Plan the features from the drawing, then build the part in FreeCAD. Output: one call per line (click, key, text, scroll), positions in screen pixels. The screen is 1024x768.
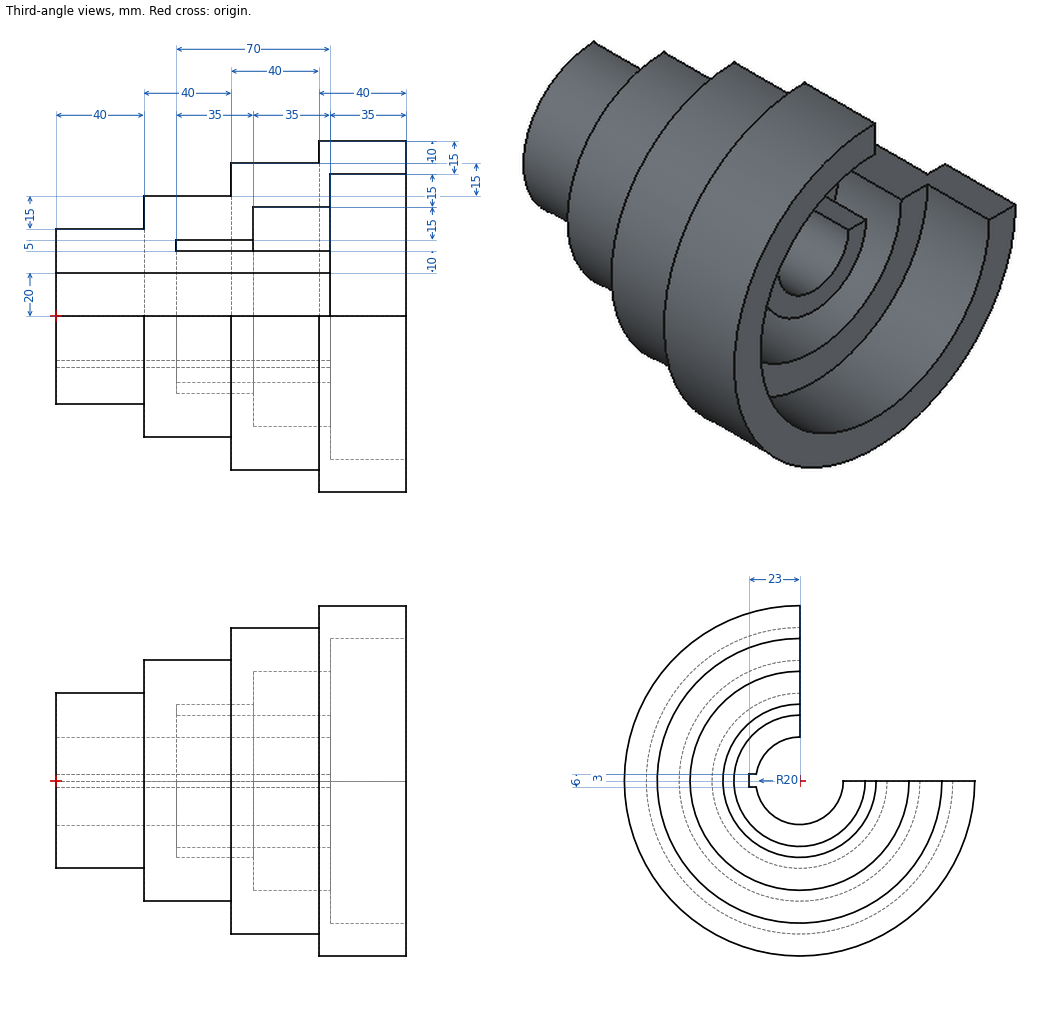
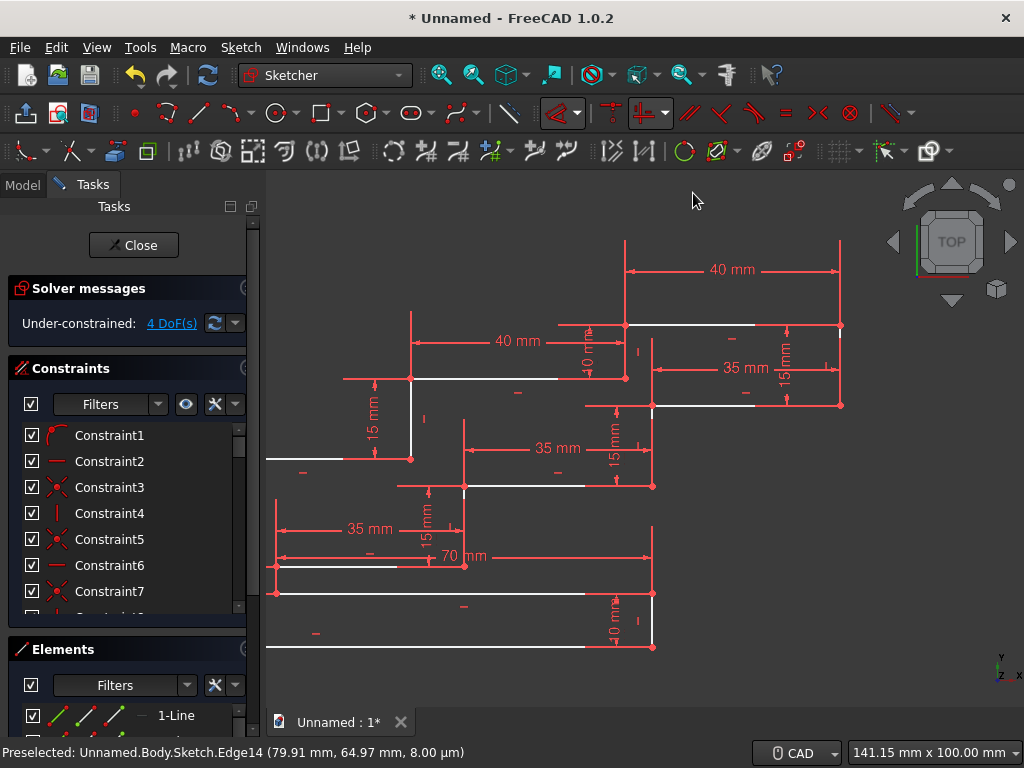
click(346, 459)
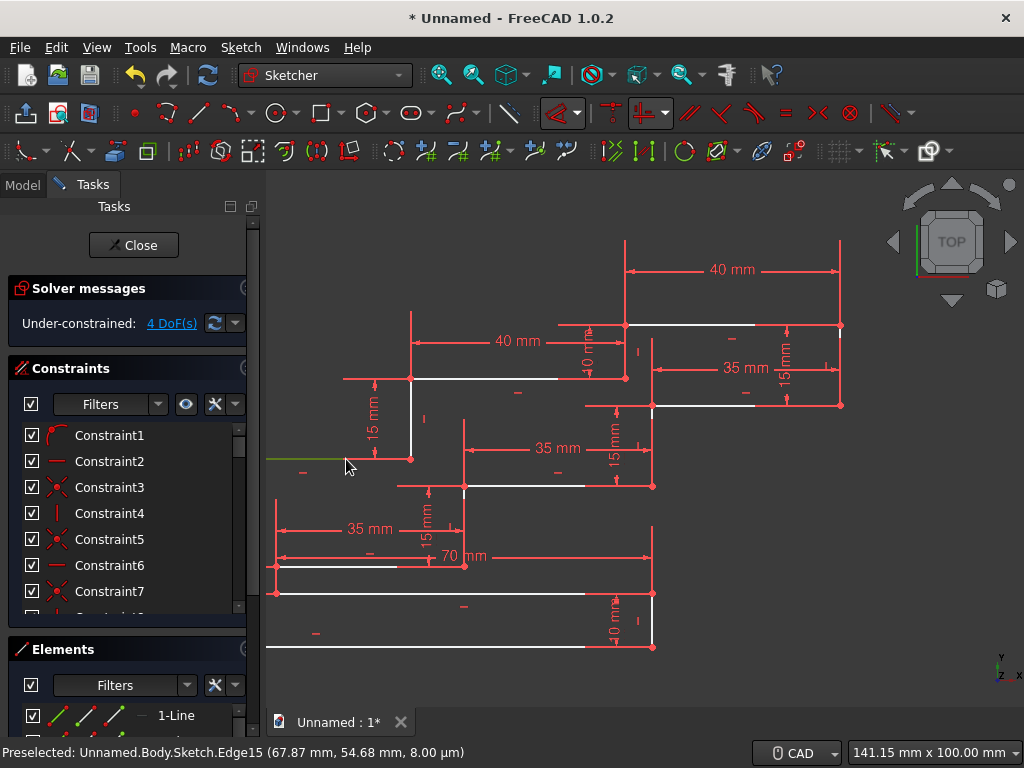
key(l)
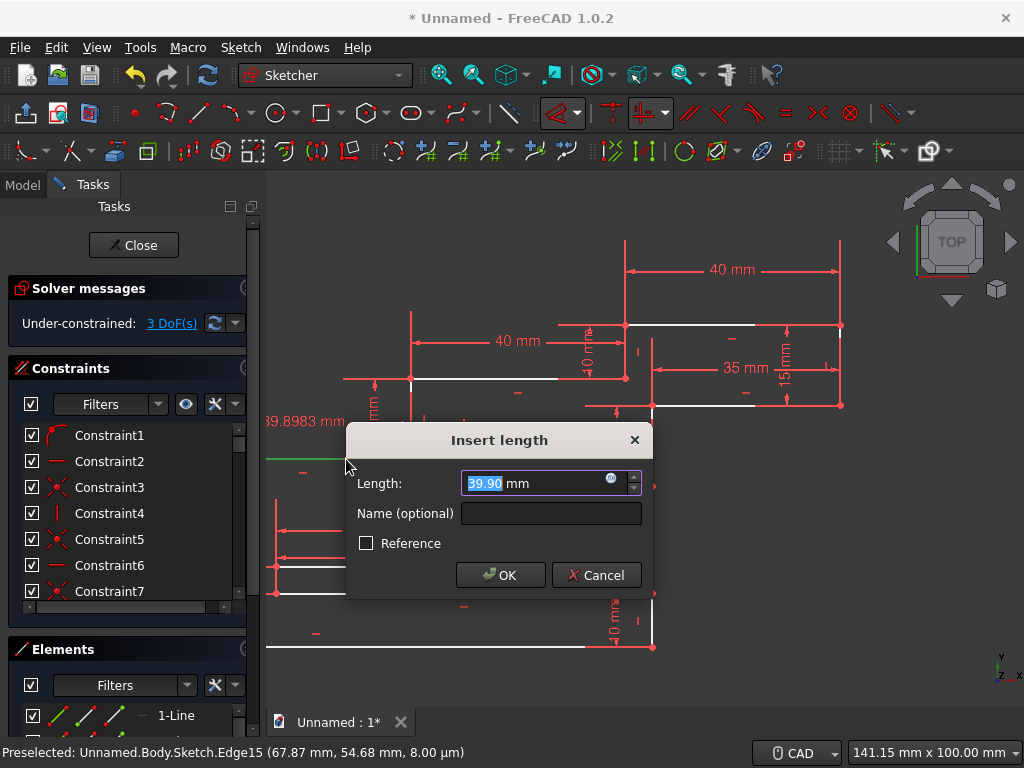
text(40)
key(Return)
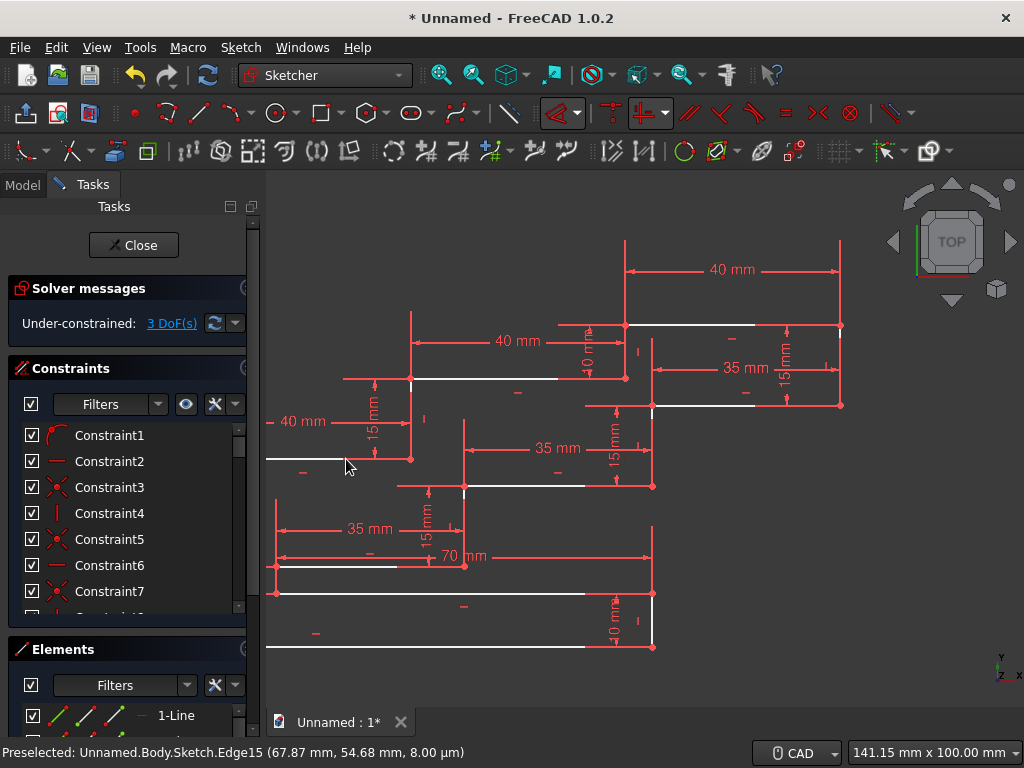
scroll(711, 357, down, 4)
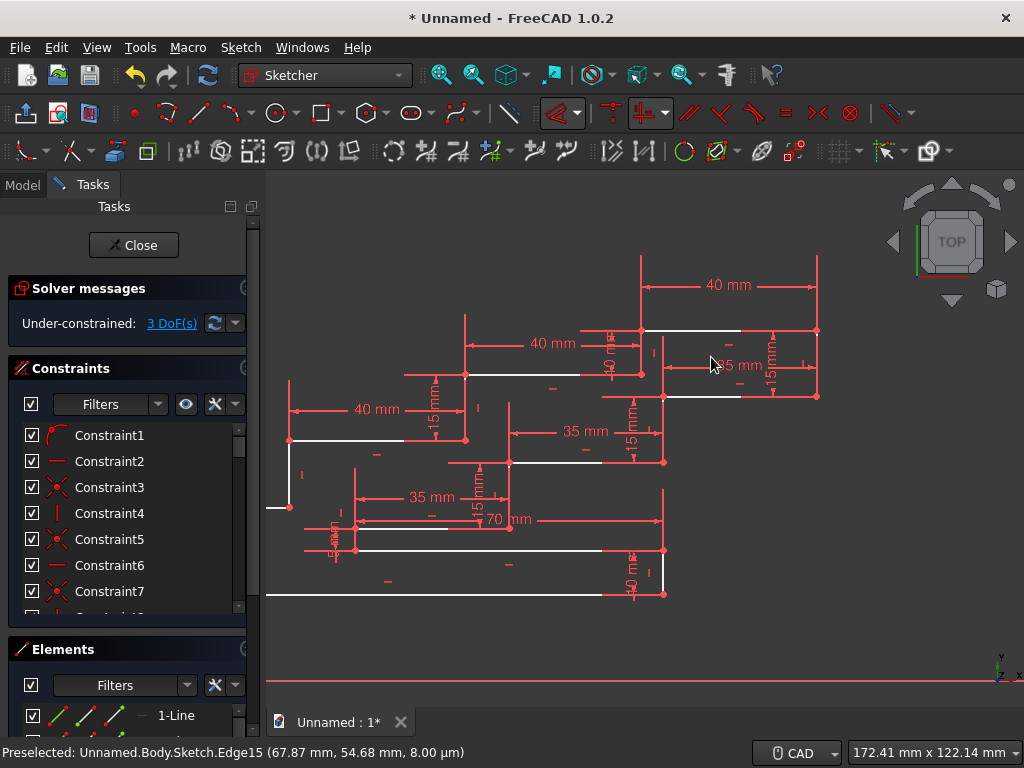
scroll(480, 414, up, 2)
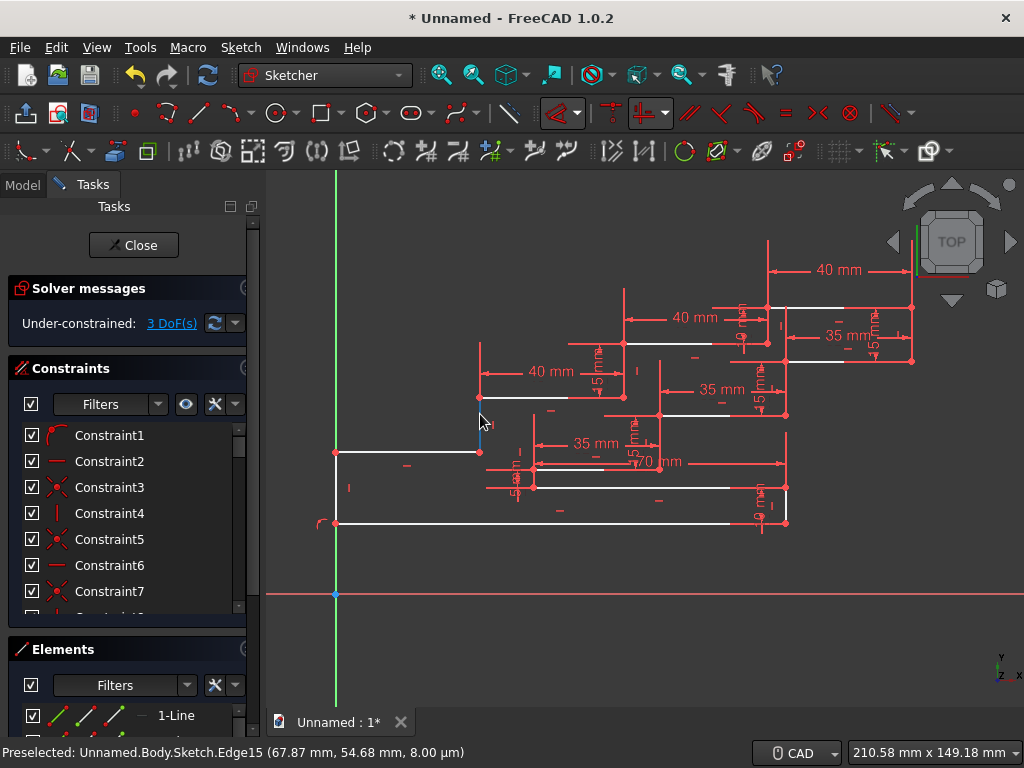
click(480, 414)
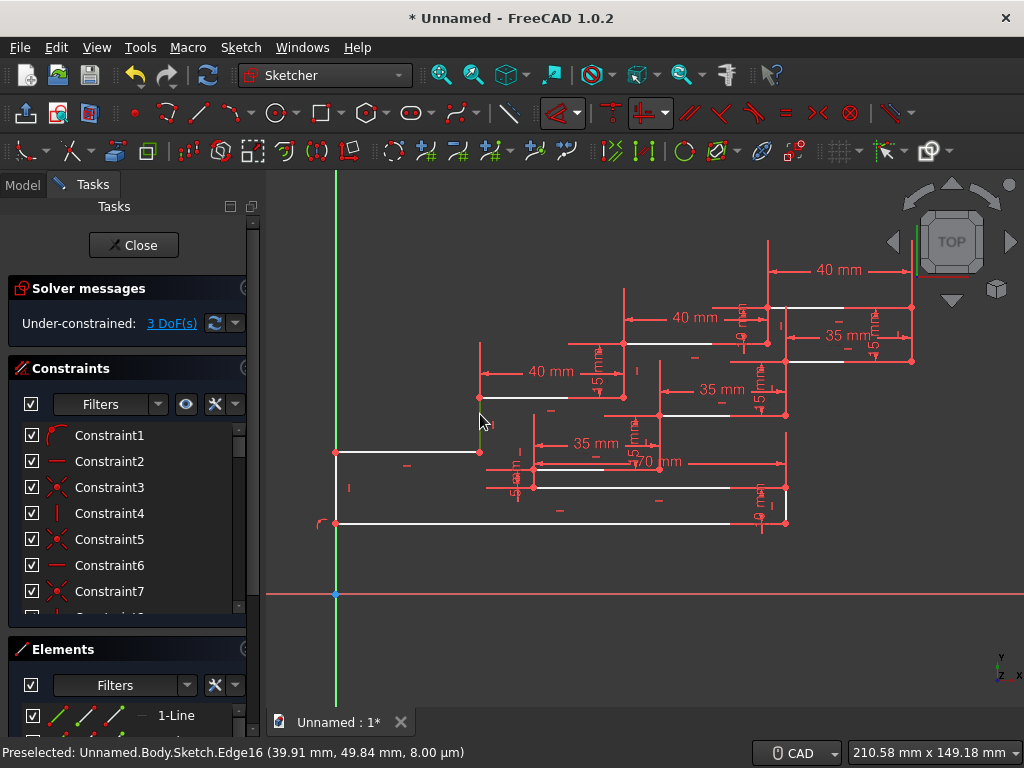
key(i)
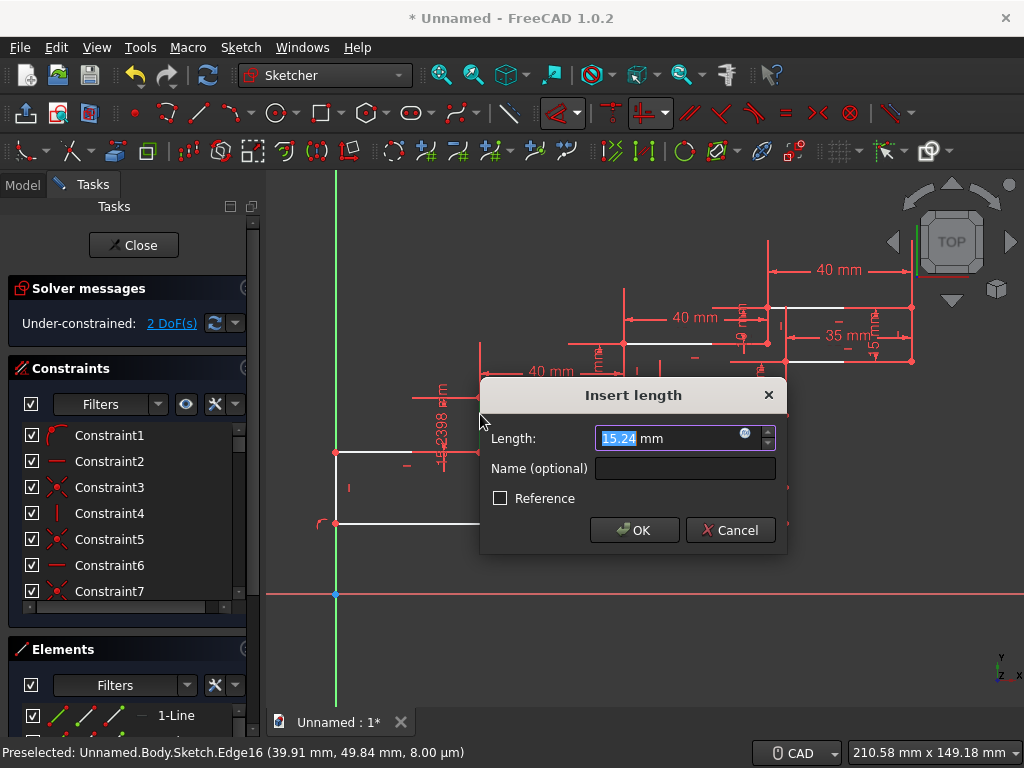
text(15)
key(Return)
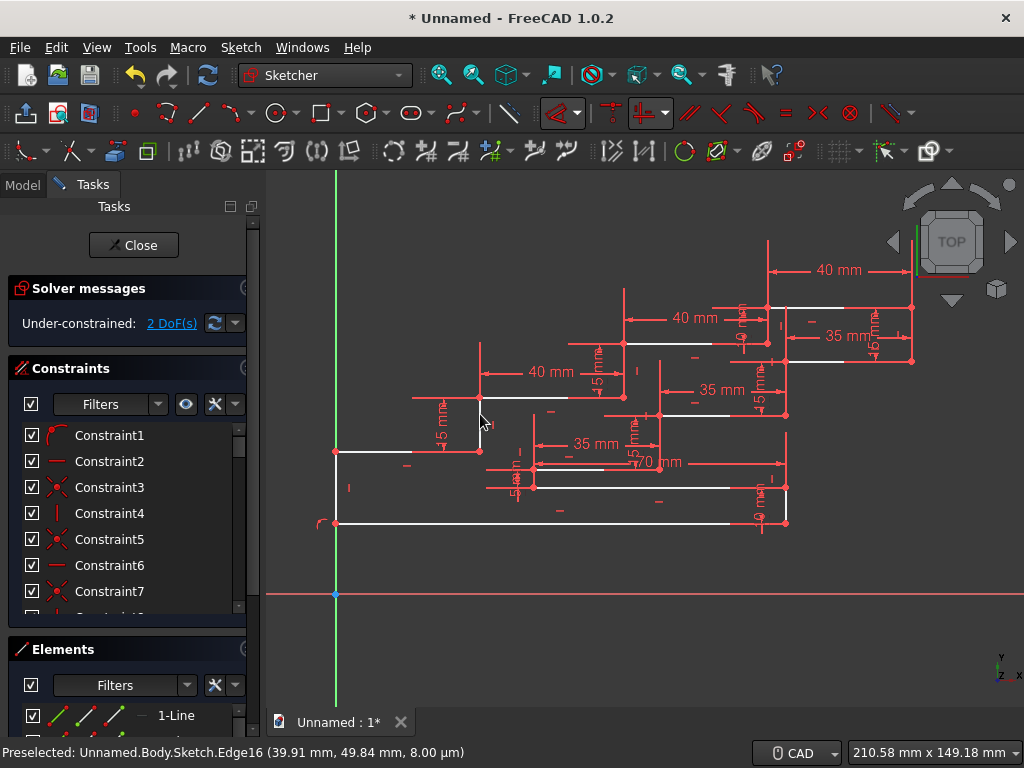
click(437, 452)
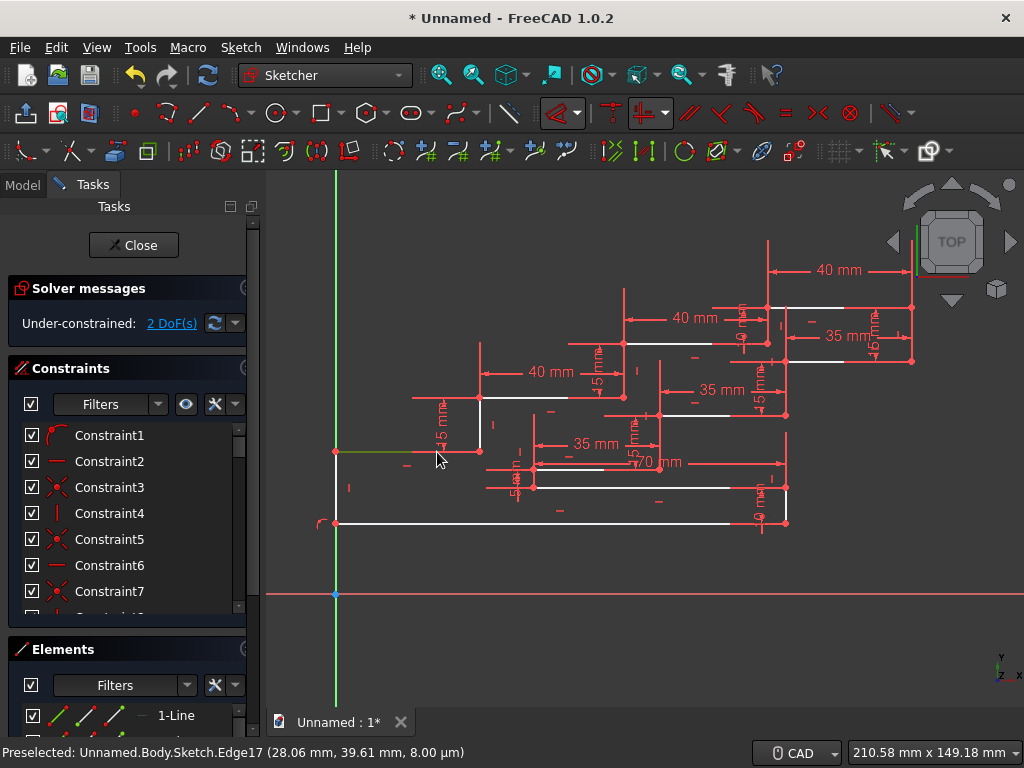
click(580, 114)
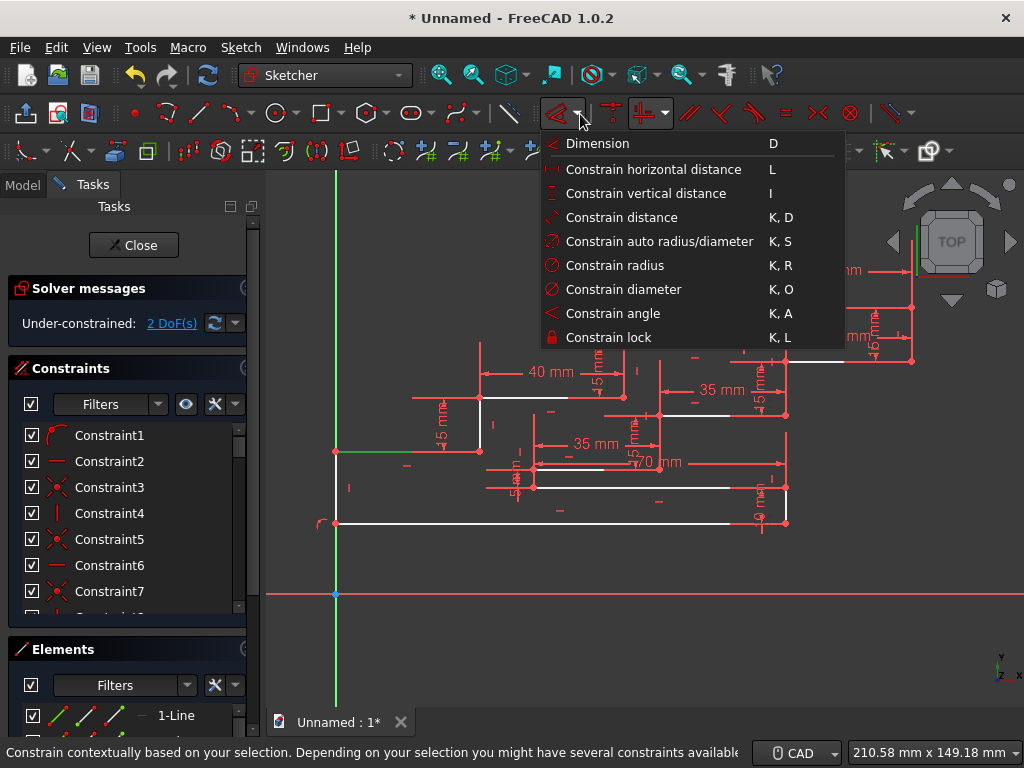
click(693, 169)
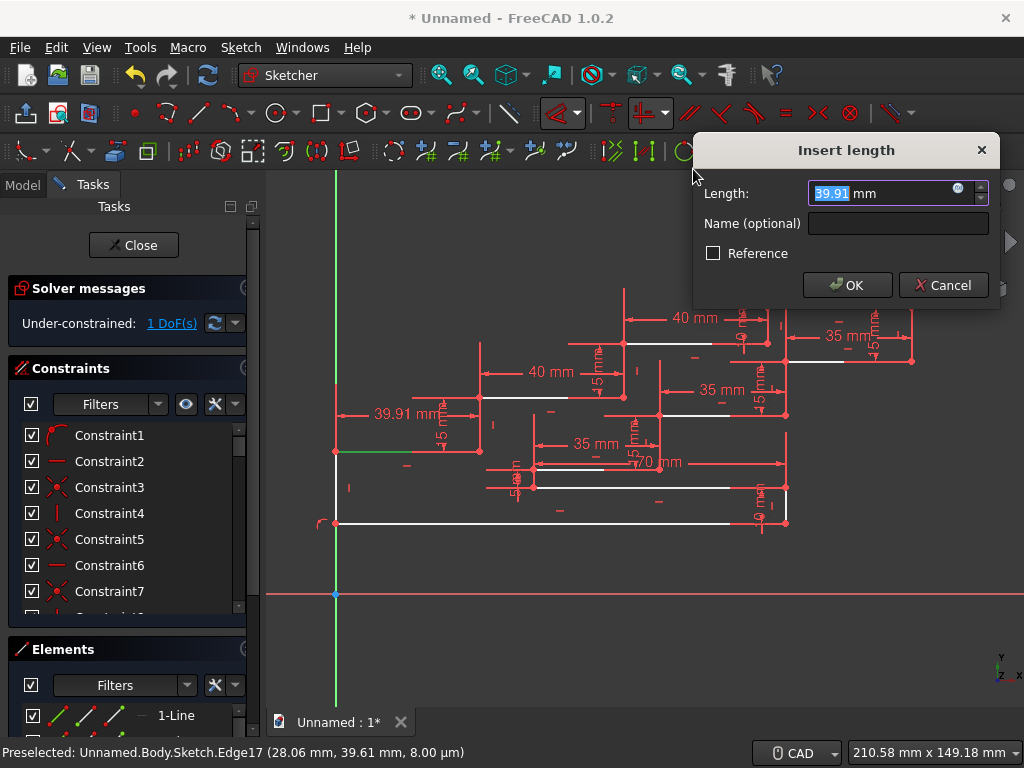
text(40)
key(Return)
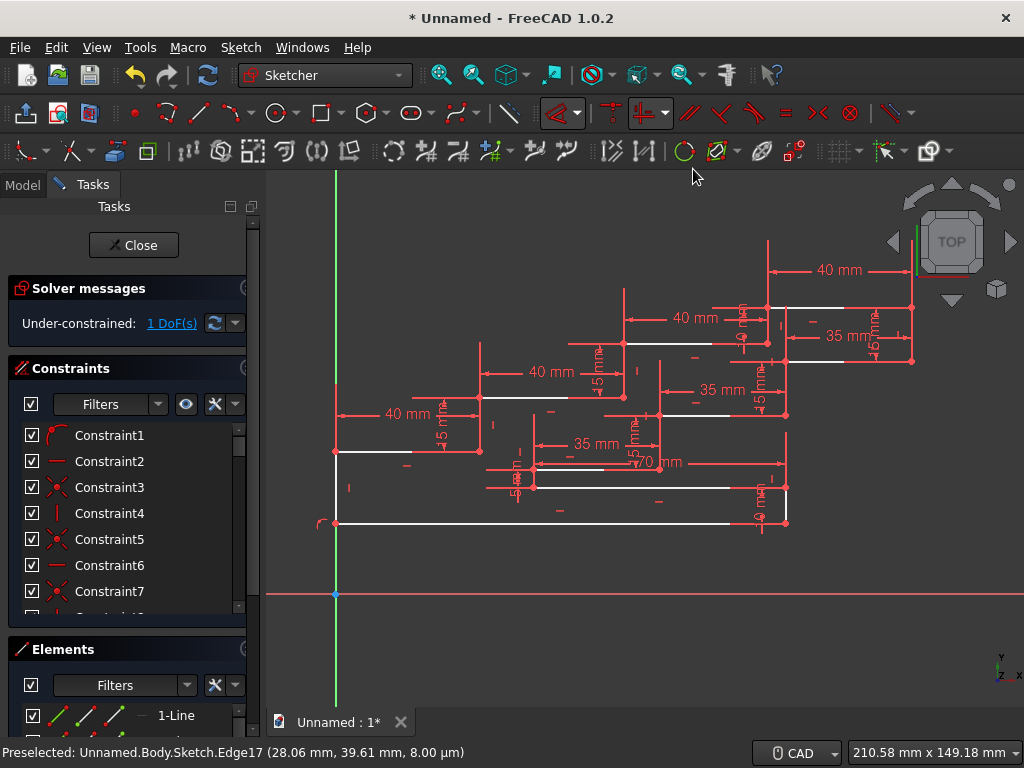
click(336, 524)